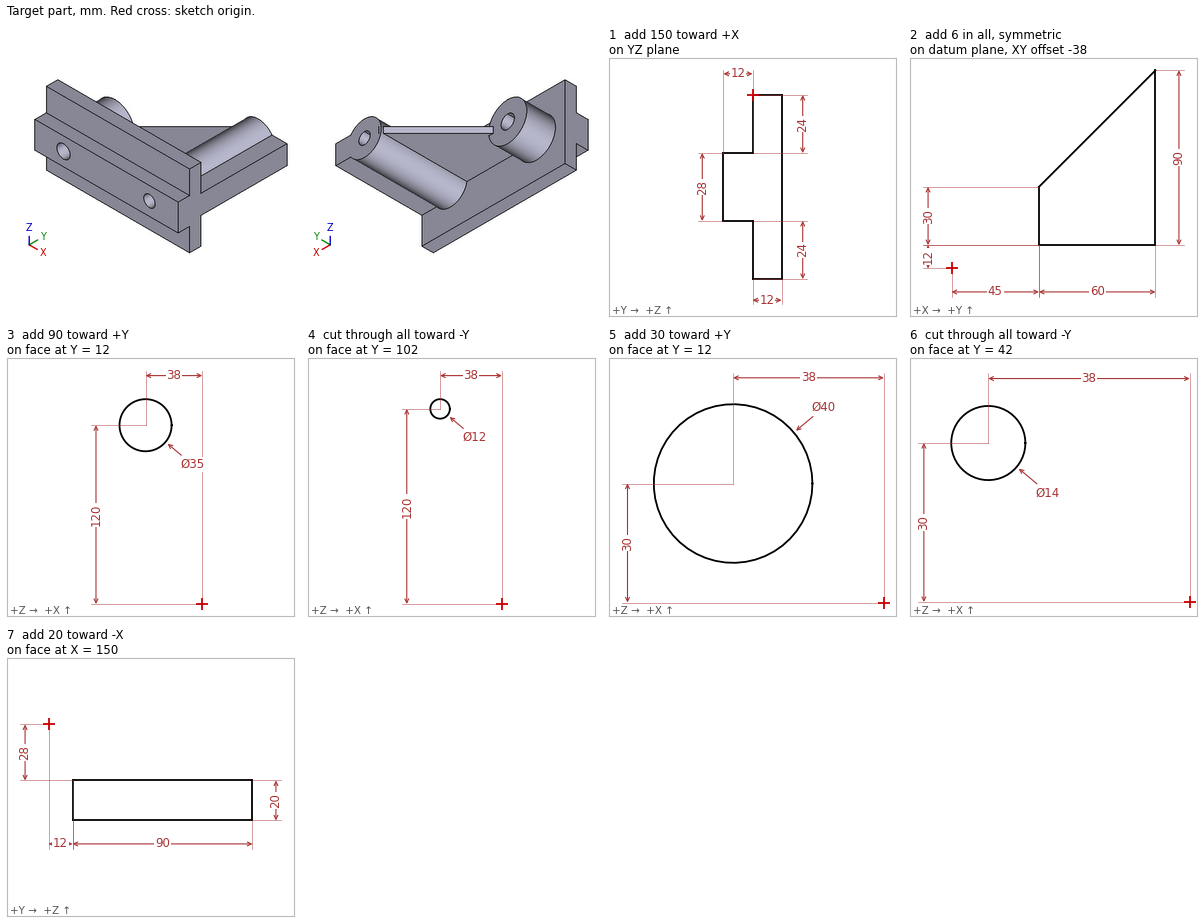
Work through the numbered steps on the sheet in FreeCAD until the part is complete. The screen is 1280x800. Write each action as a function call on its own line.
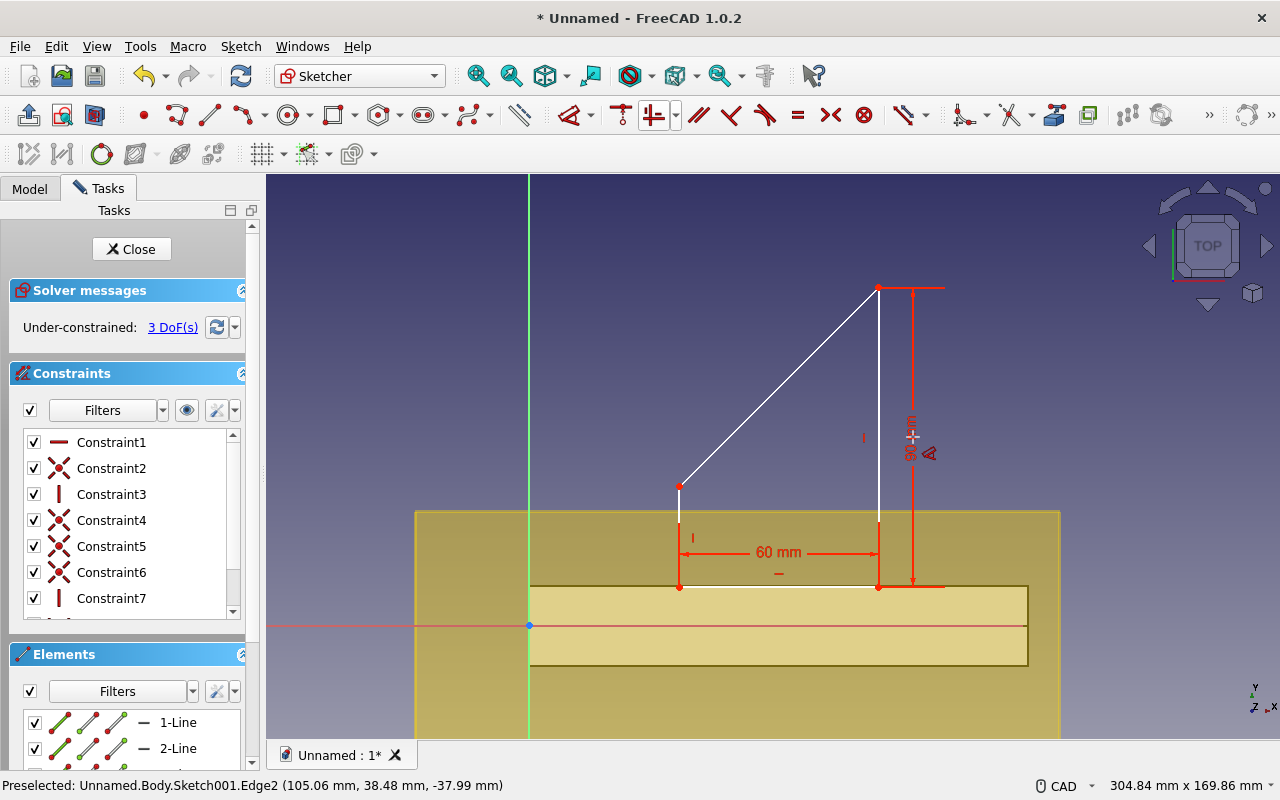
click(679, 517)
click(645, 537)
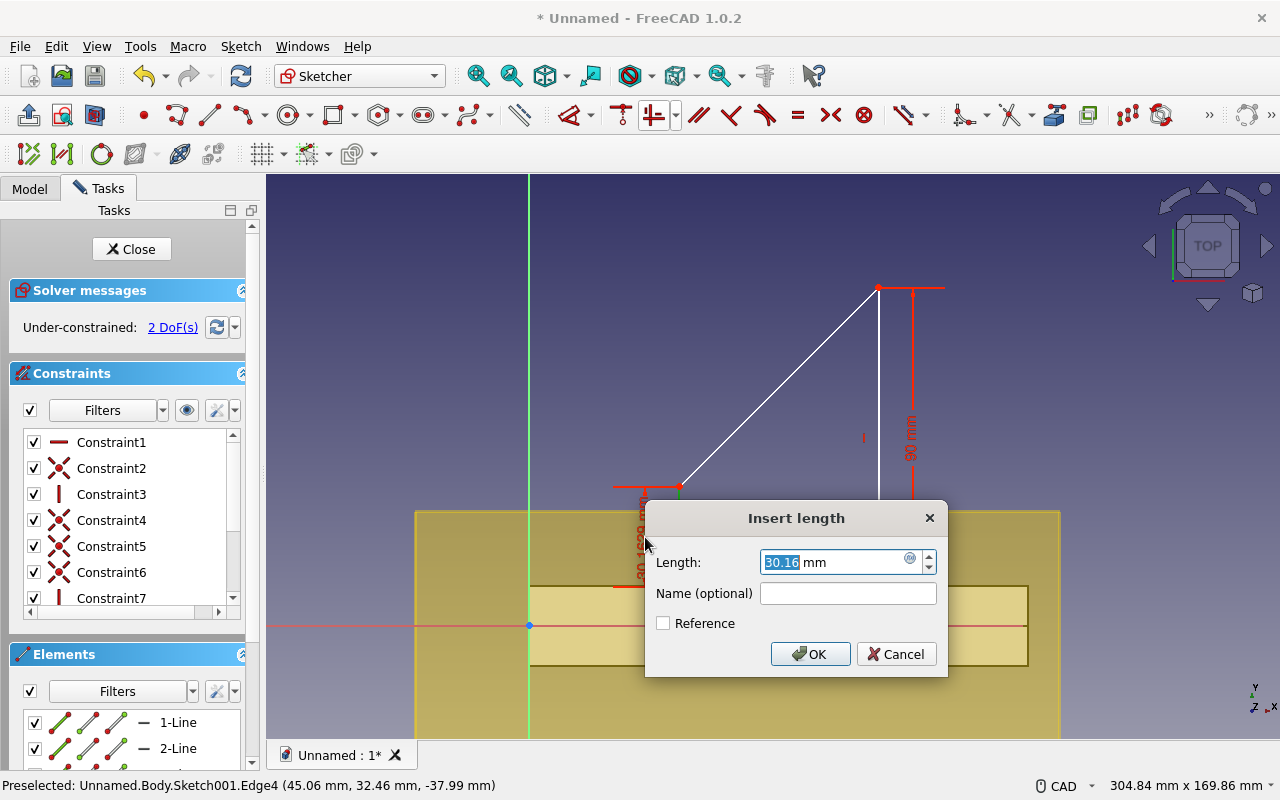
text(30)
key(Return)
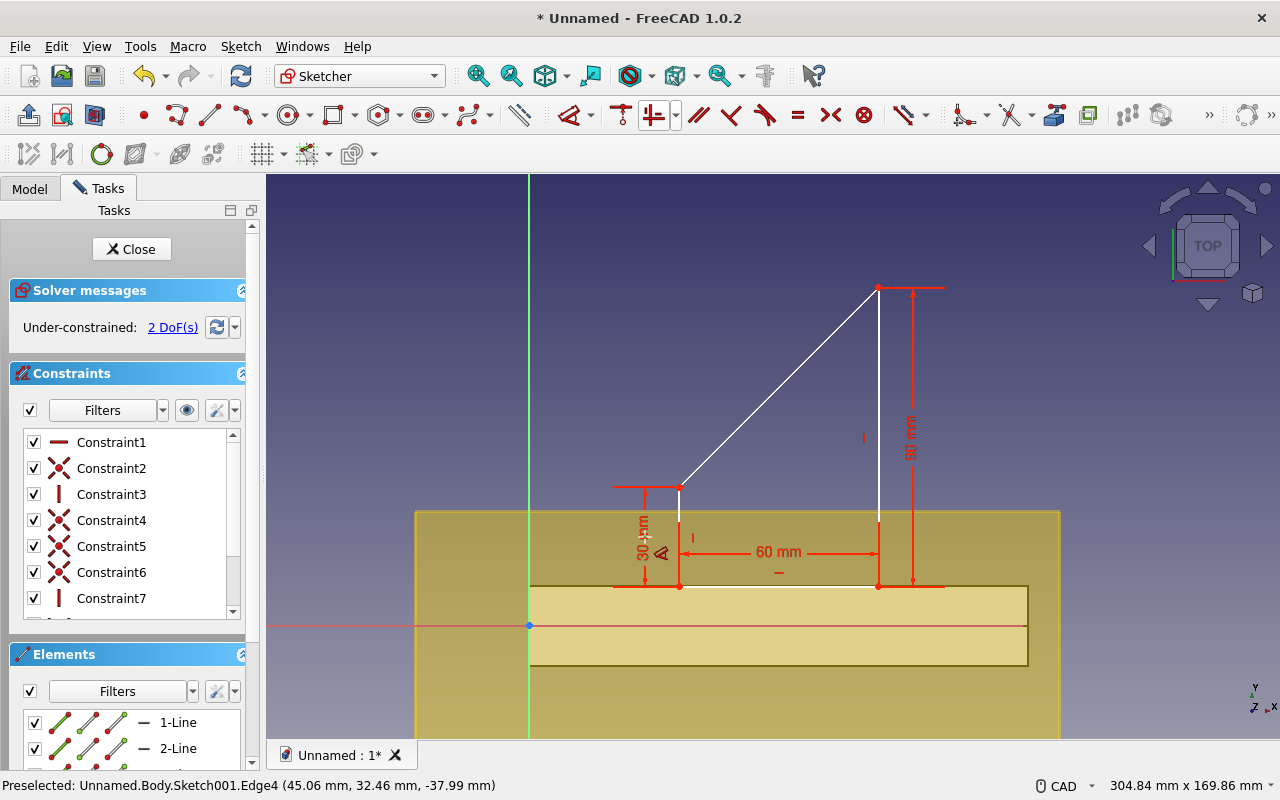
click(679, 587)
click(604, 660)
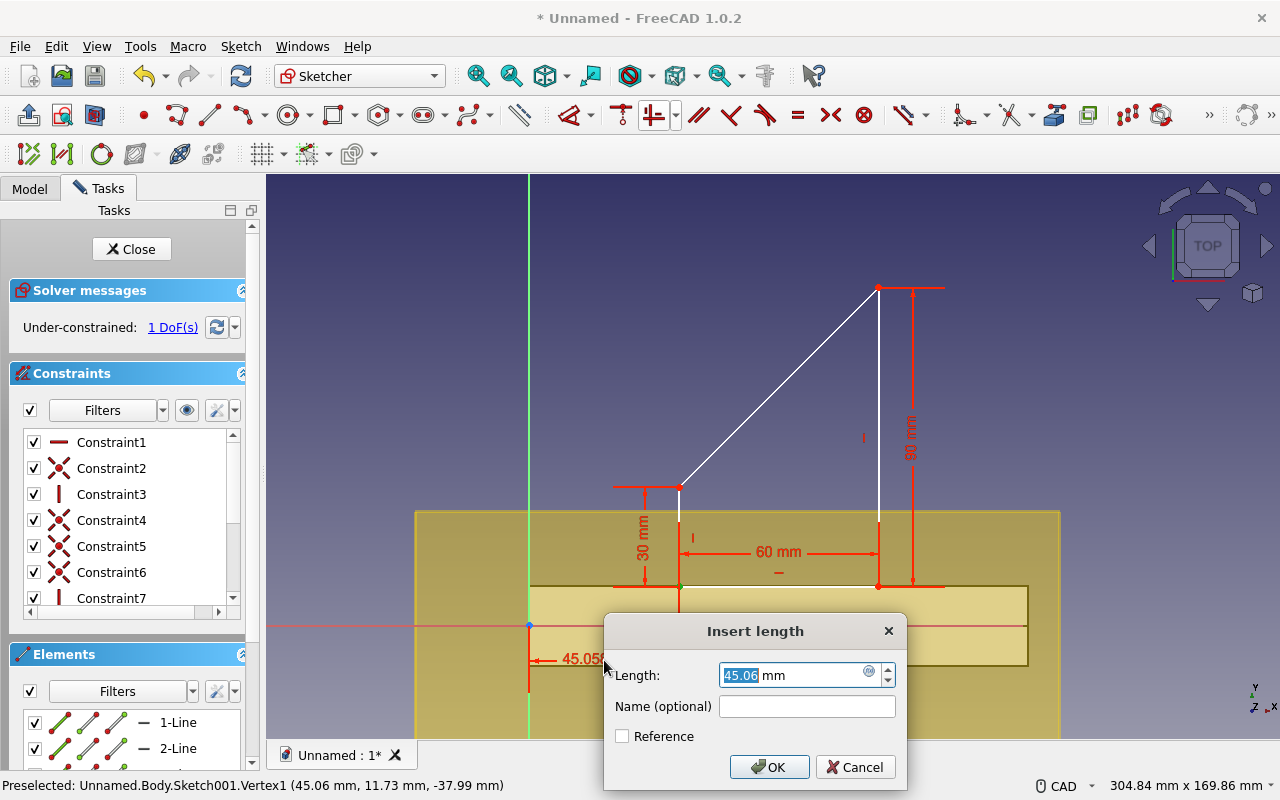
text(45)
key(Return)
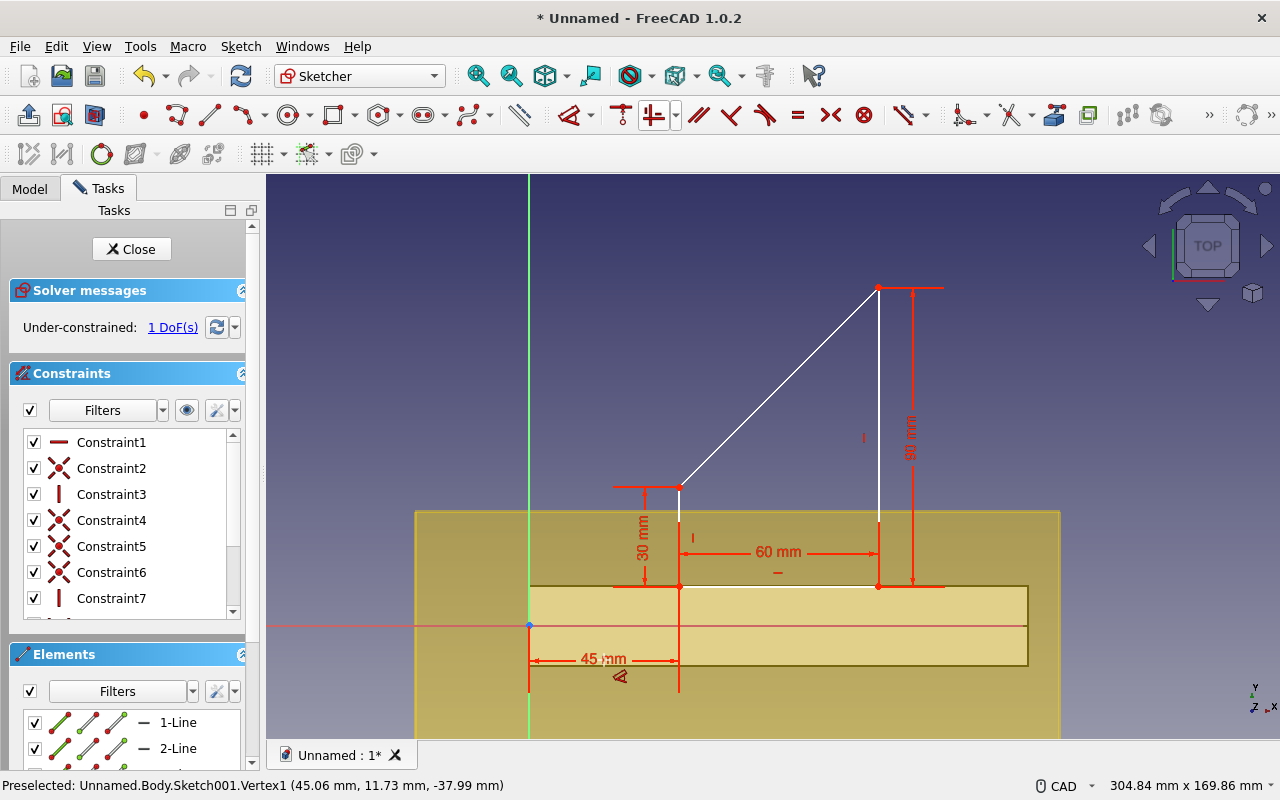
click(679, 587)
click(495, 606)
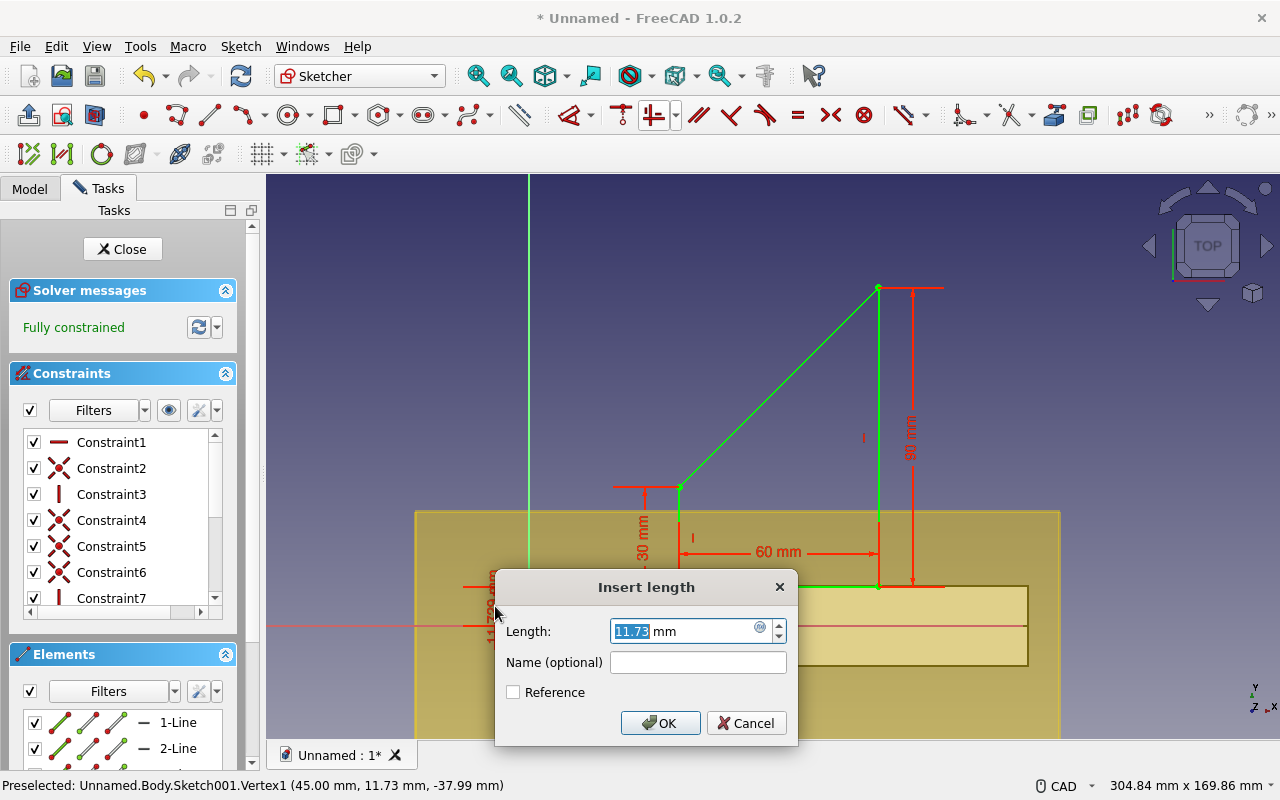
text(12)
key(Return)
key(Escape)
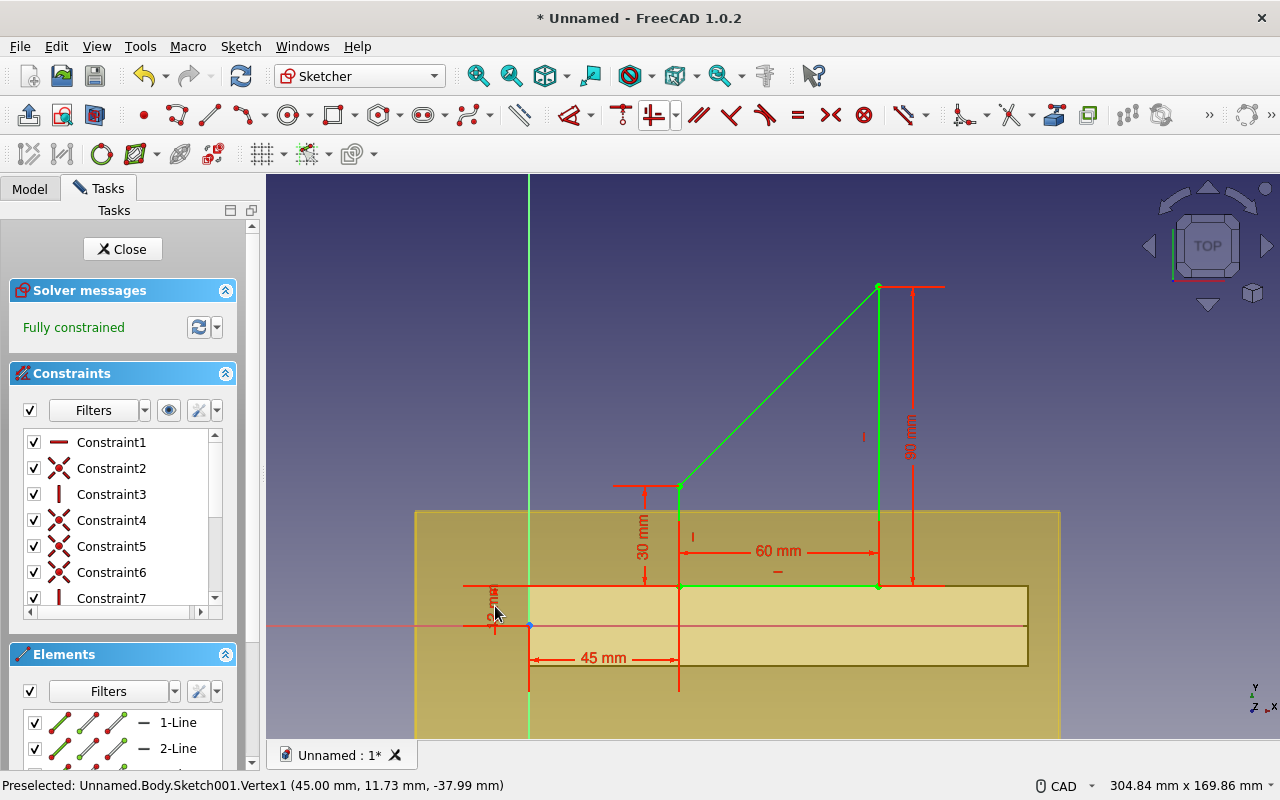
click(123, 249)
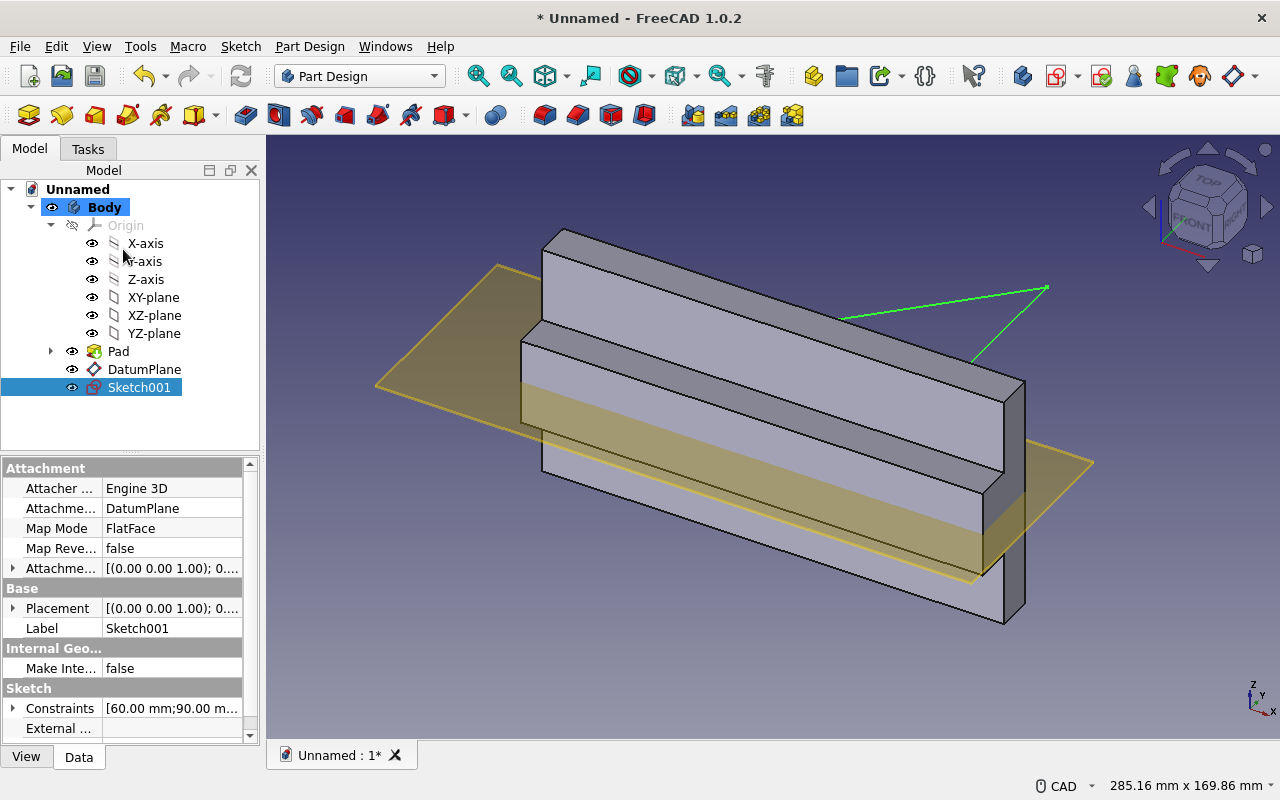
click(29, 116)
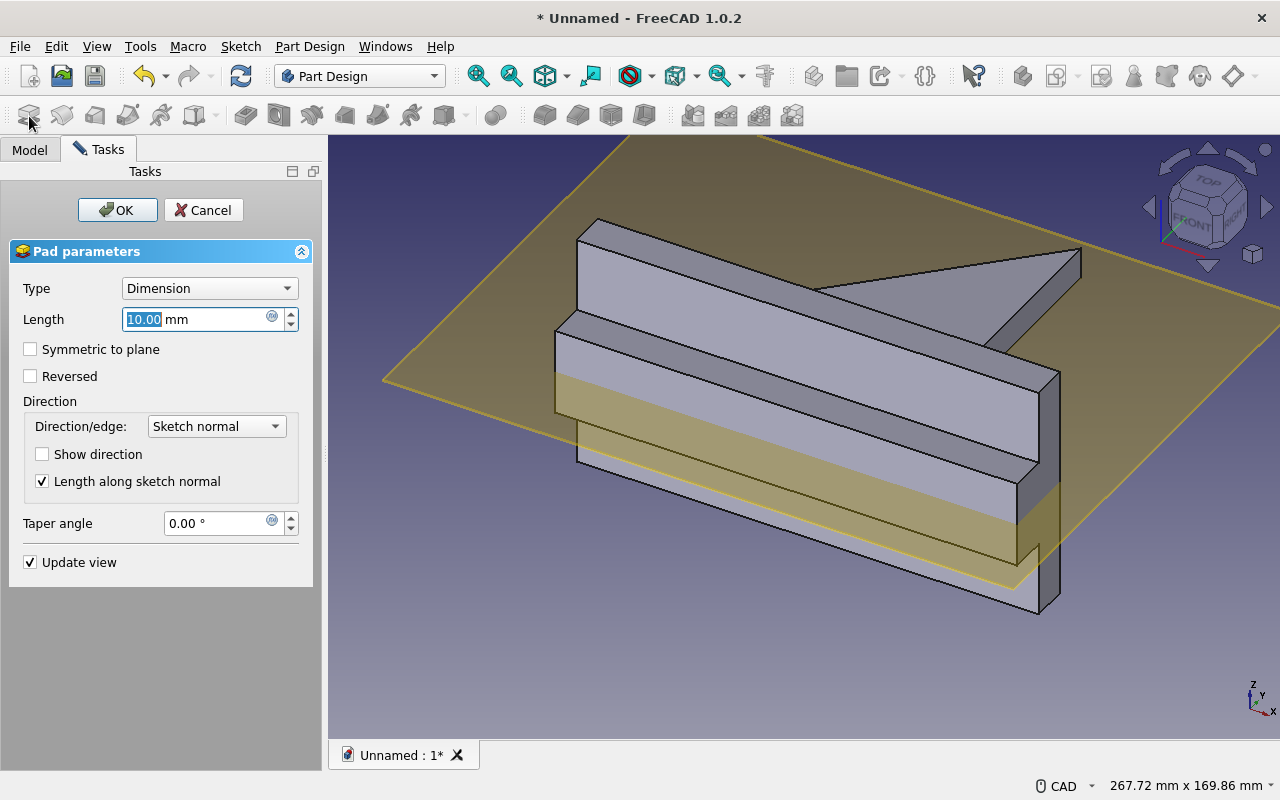
text(6)
key(Tab)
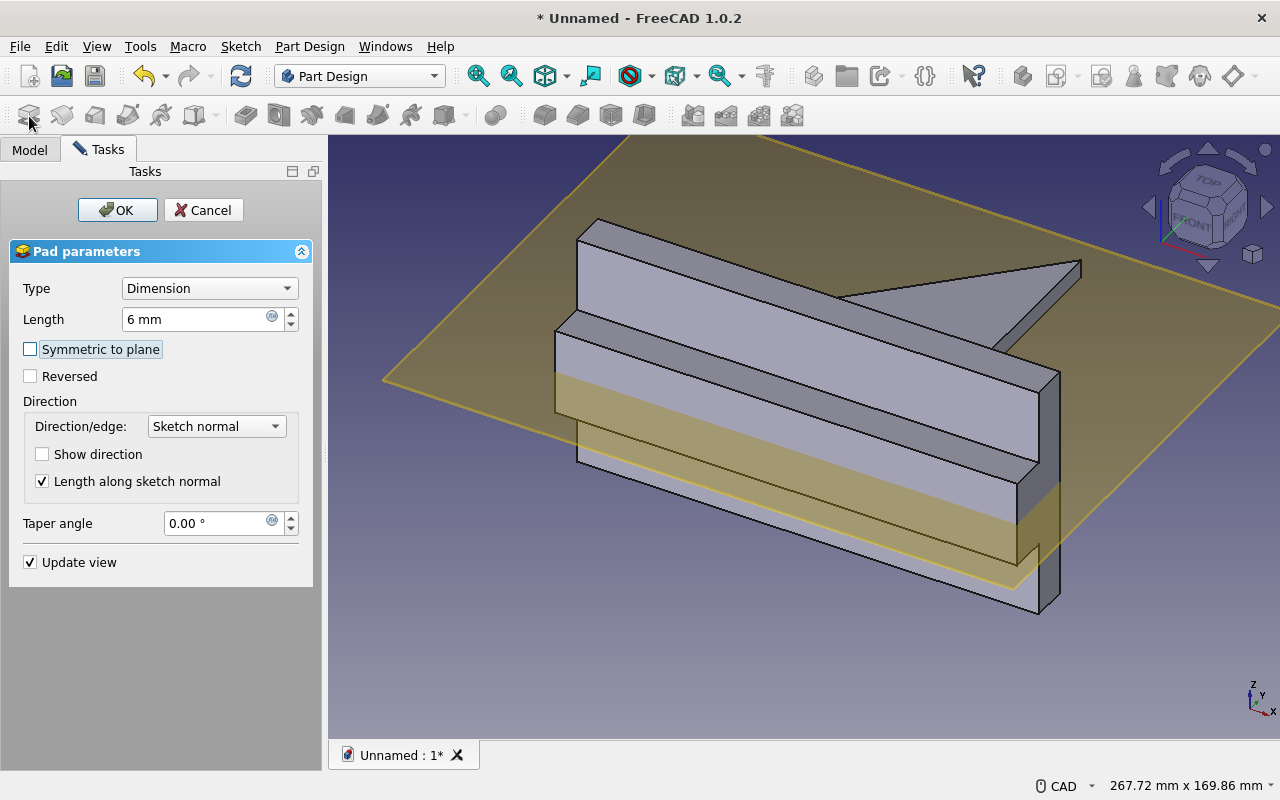
click(31, 349)